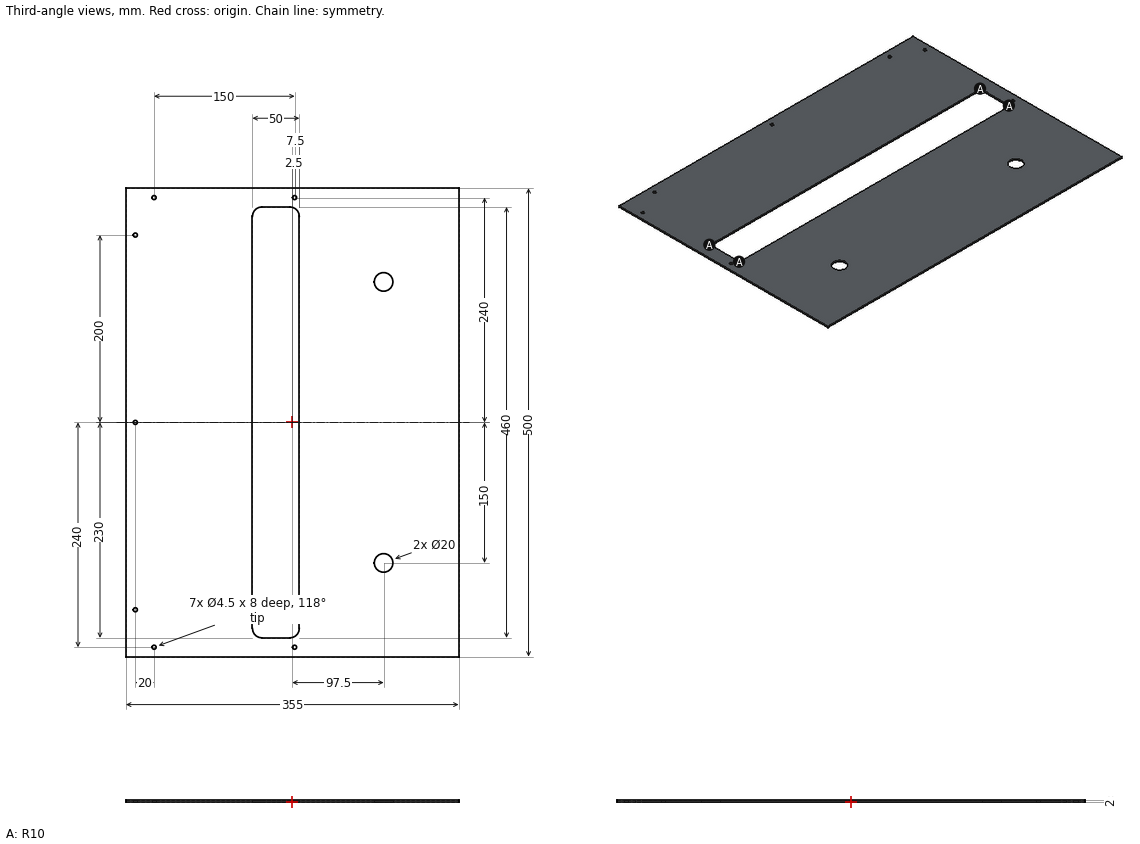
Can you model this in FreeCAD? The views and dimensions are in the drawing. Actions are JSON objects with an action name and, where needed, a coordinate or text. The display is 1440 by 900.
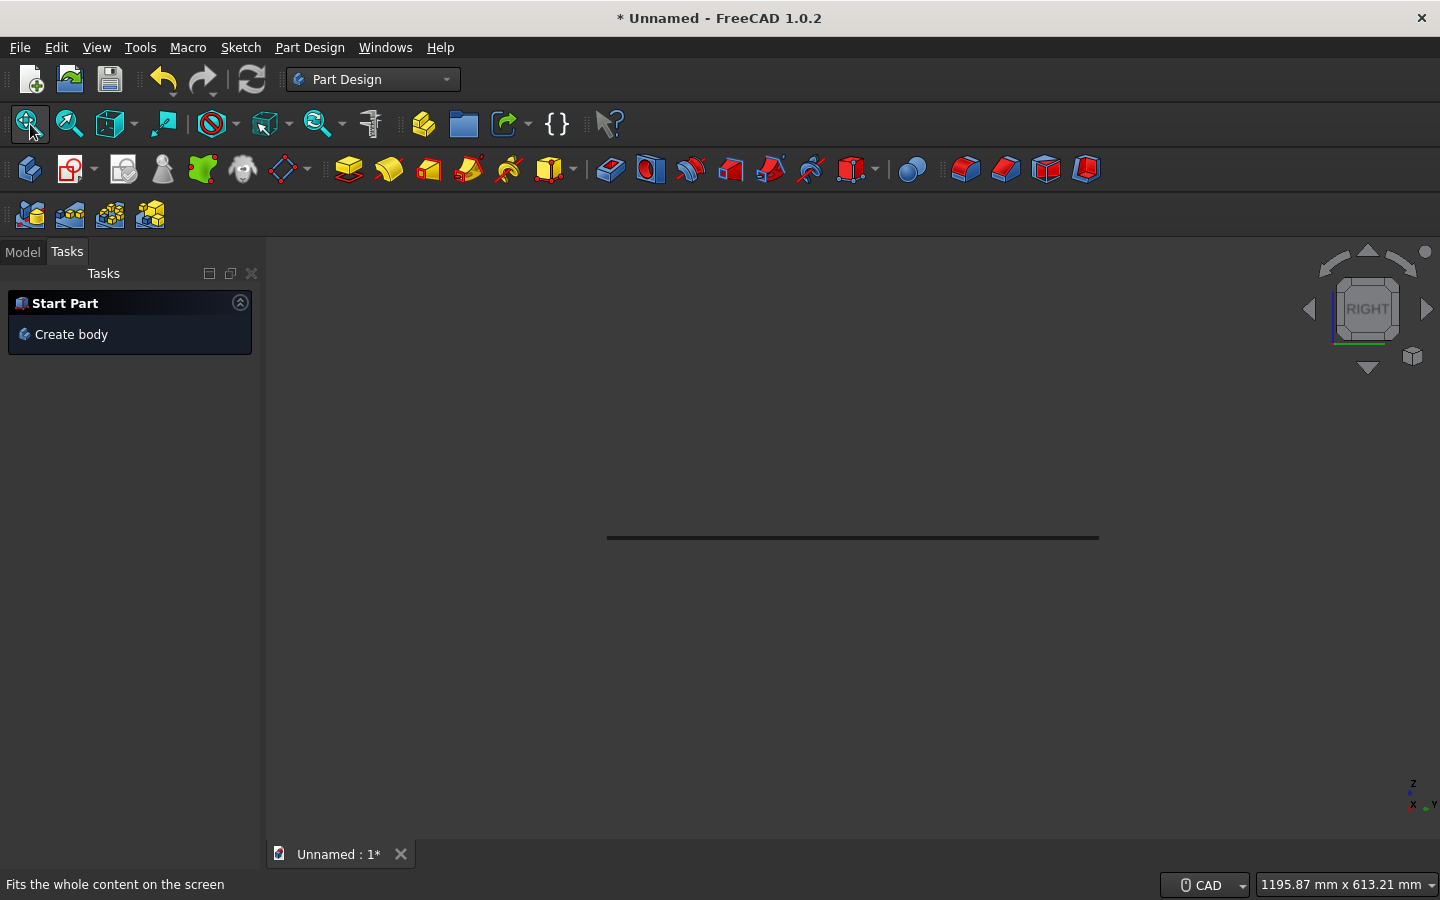
{"action": "key", "text": "5"}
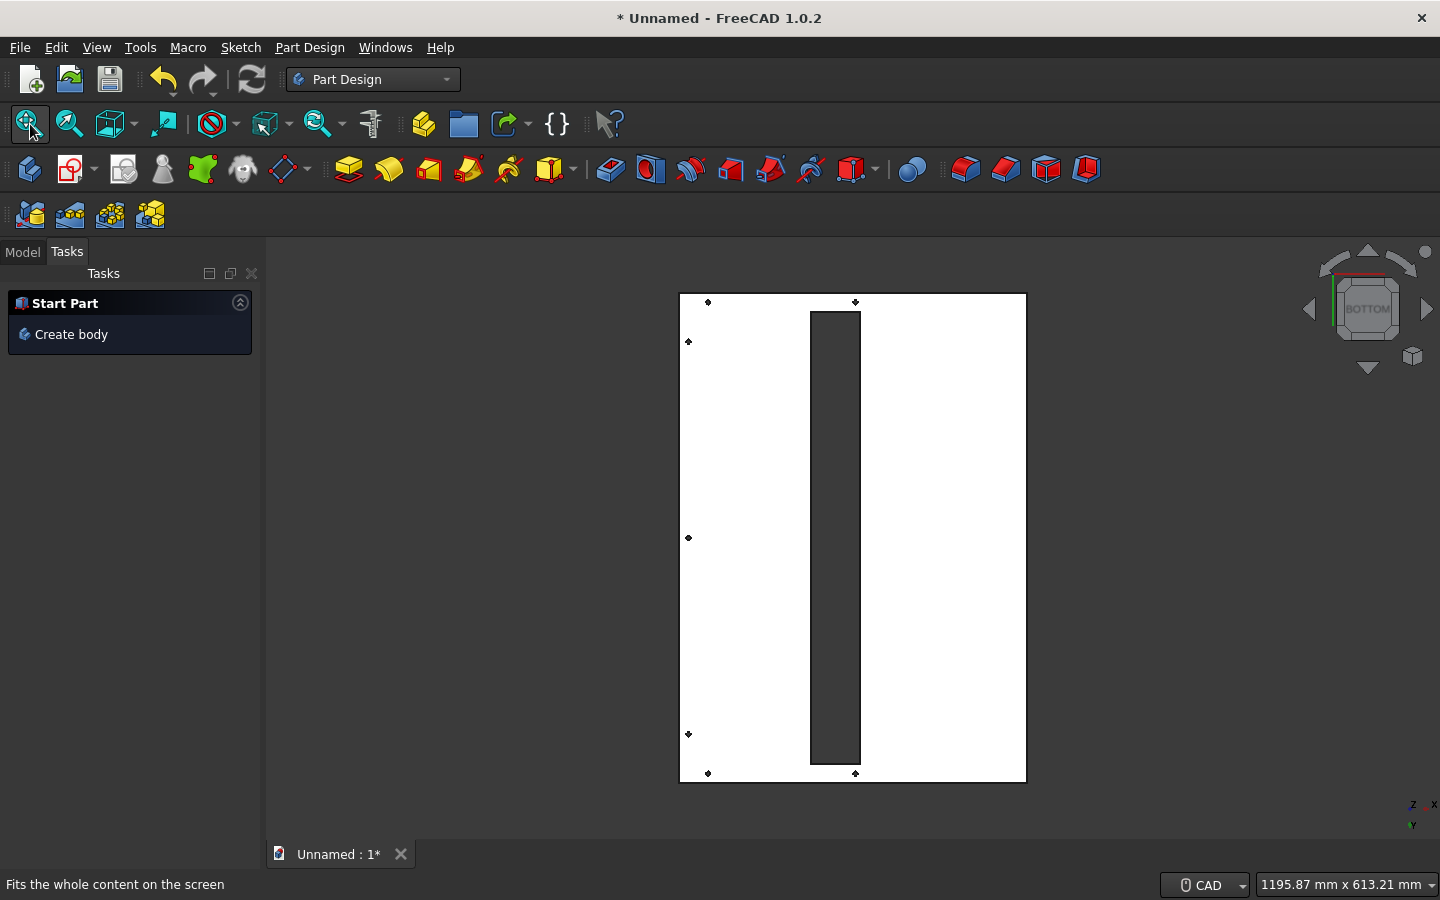
{"action": "scroll", "coordinate": [811, 763], "scroll_direction": "up", "scroll_amount": 15}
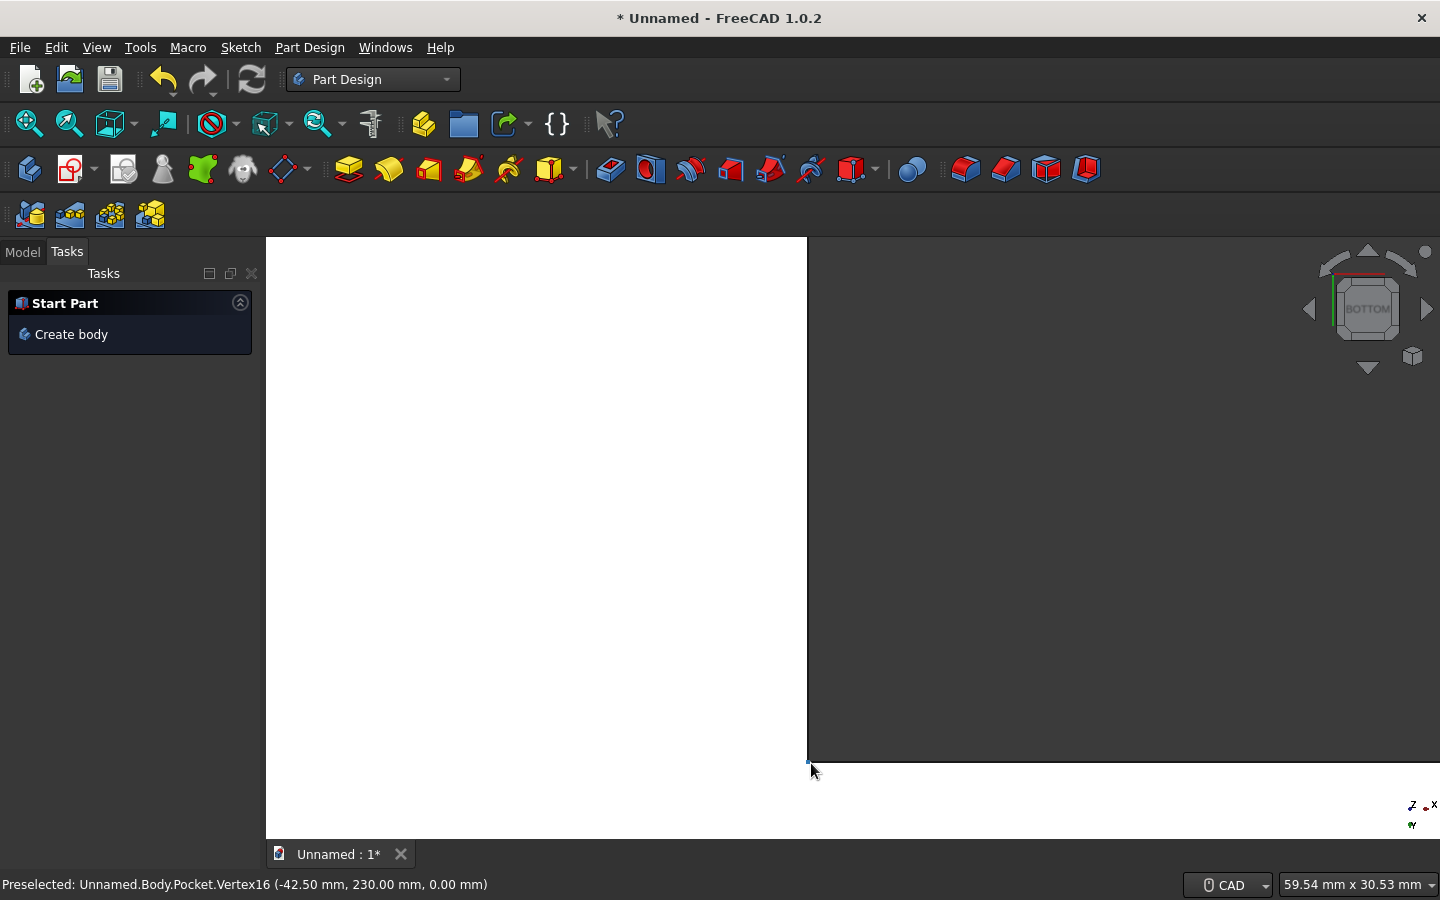
{"action": "left_click", "coordinate": [30, 124]}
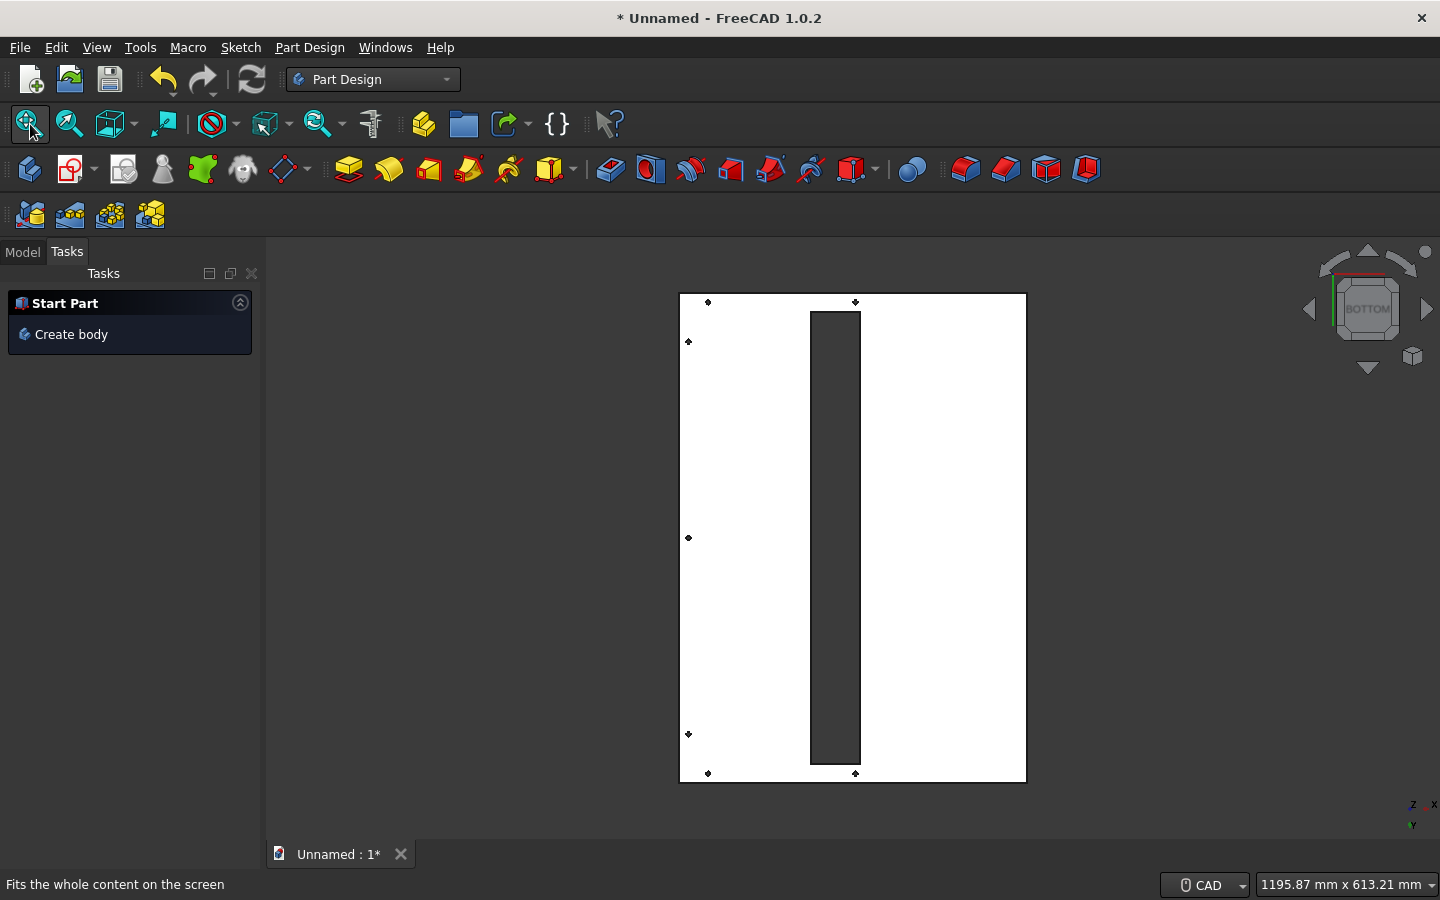
{"action": "key", "text": "4"}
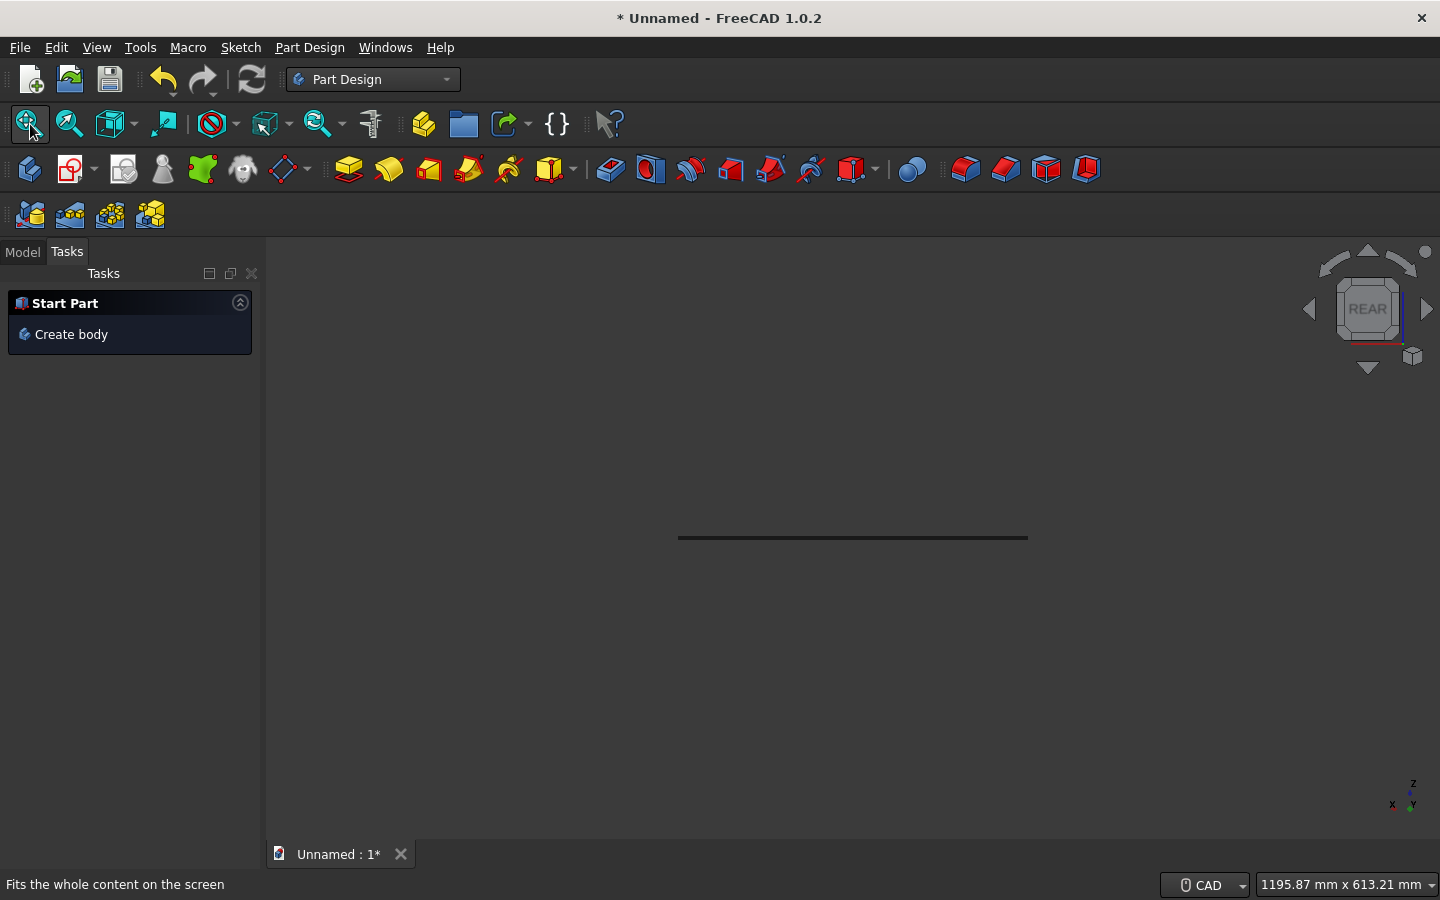
{"action": "left_click", "coordinate": [30, 124]}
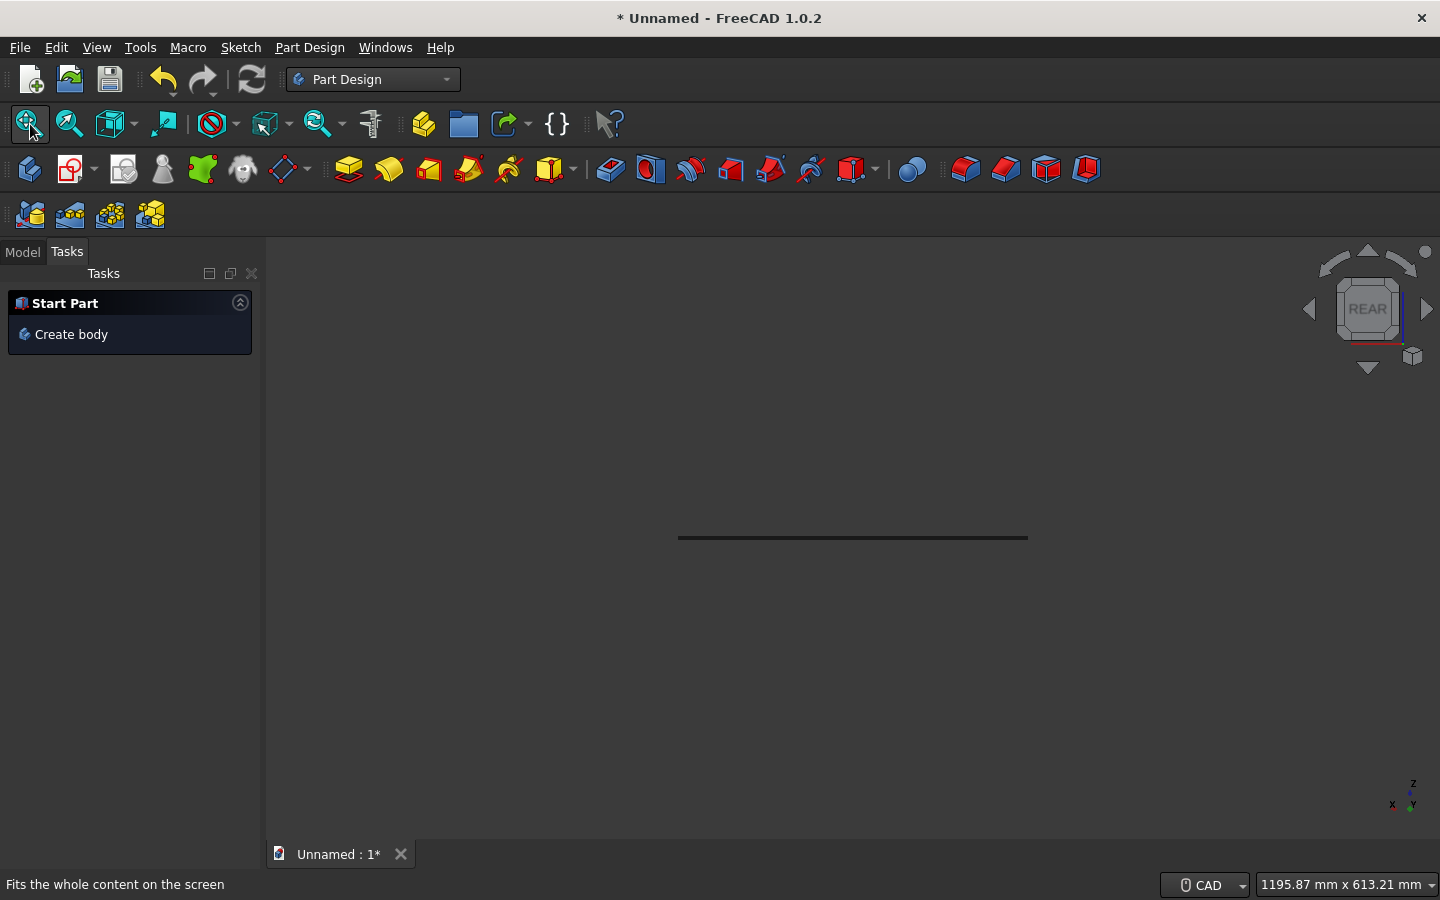
{"action": "scroll", "coordinate": [895, 537], "scroll_direction": "up", "scroll_amount": 15}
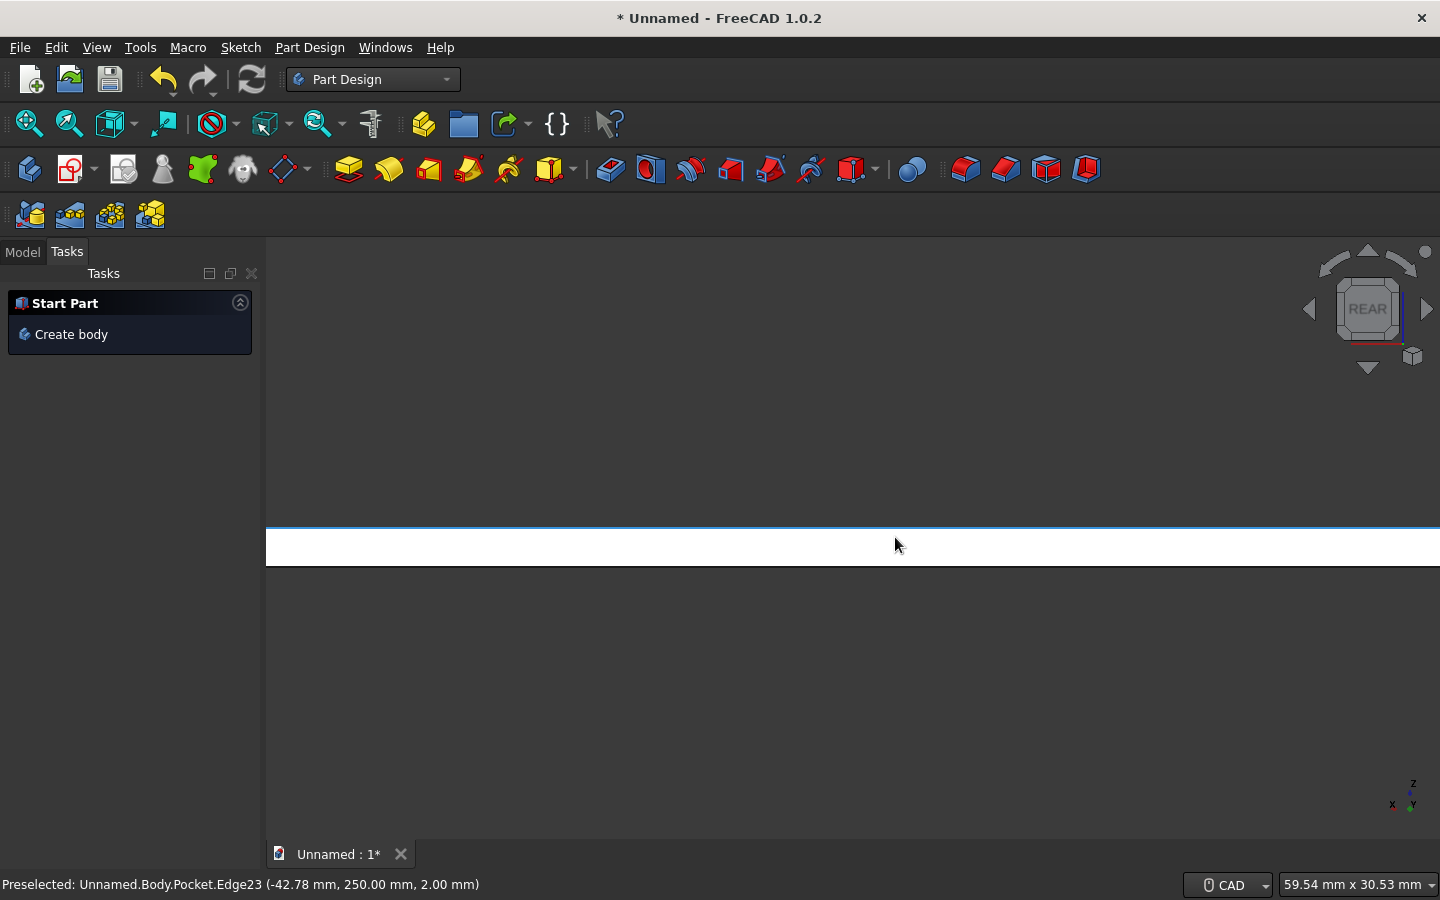
{"action": "left_click", "coordinate": [30, 124]}